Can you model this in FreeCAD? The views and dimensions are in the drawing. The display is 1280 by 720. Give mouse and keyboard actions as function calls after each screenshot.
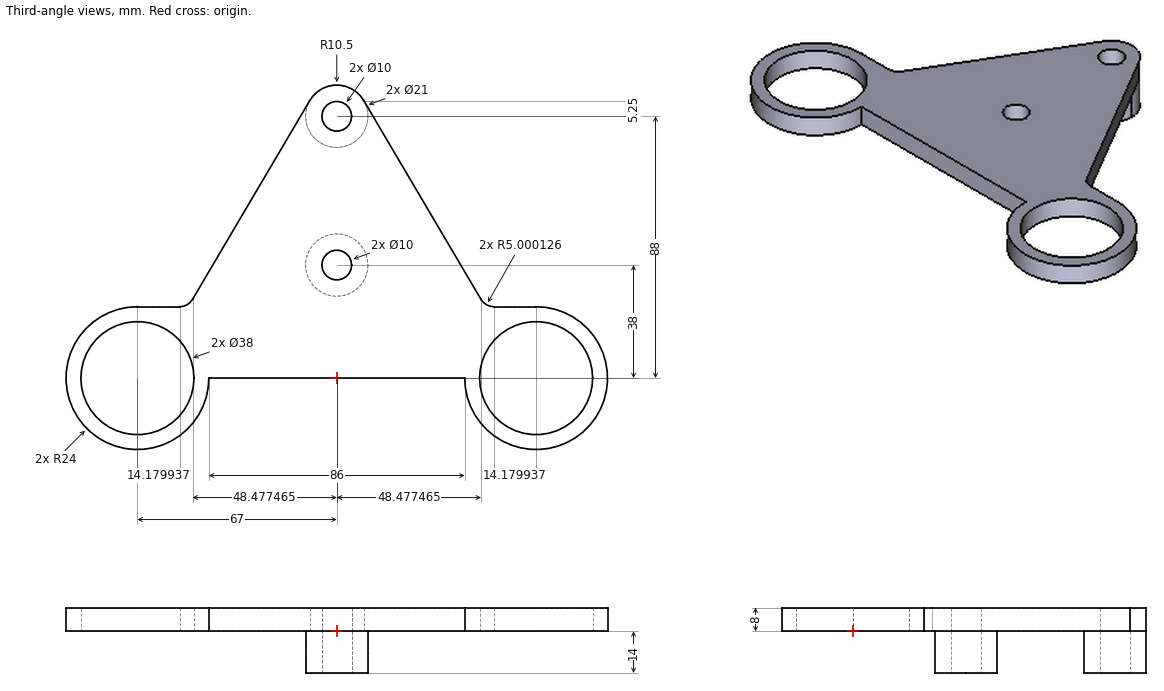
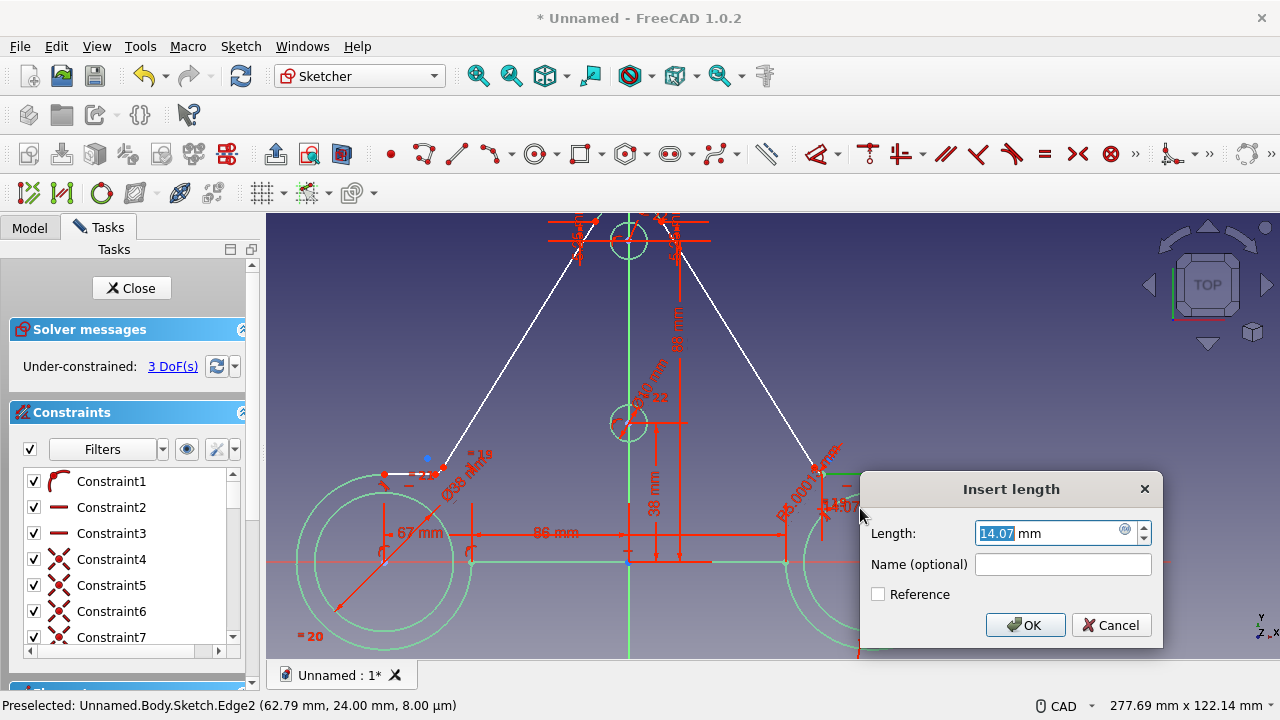
text(14.179937)
key(Return)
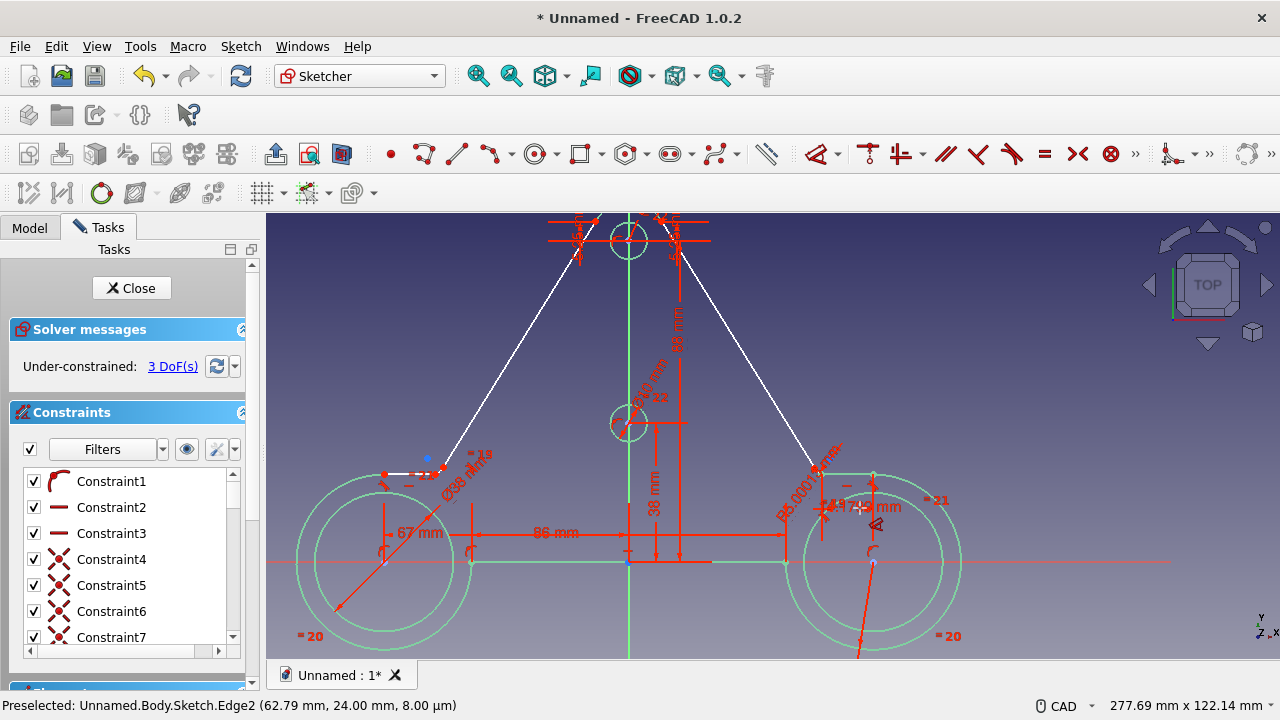
click(420, 474)
click(398, 508)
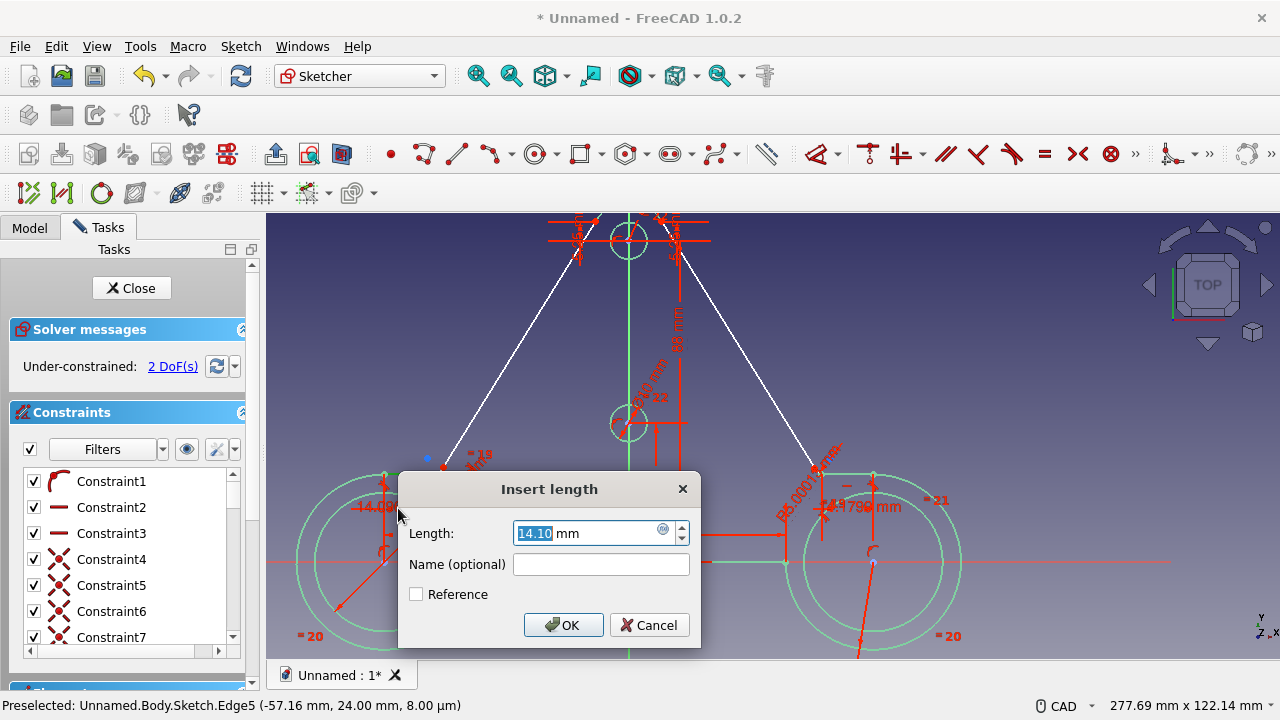
text(14.179937)
key(Return)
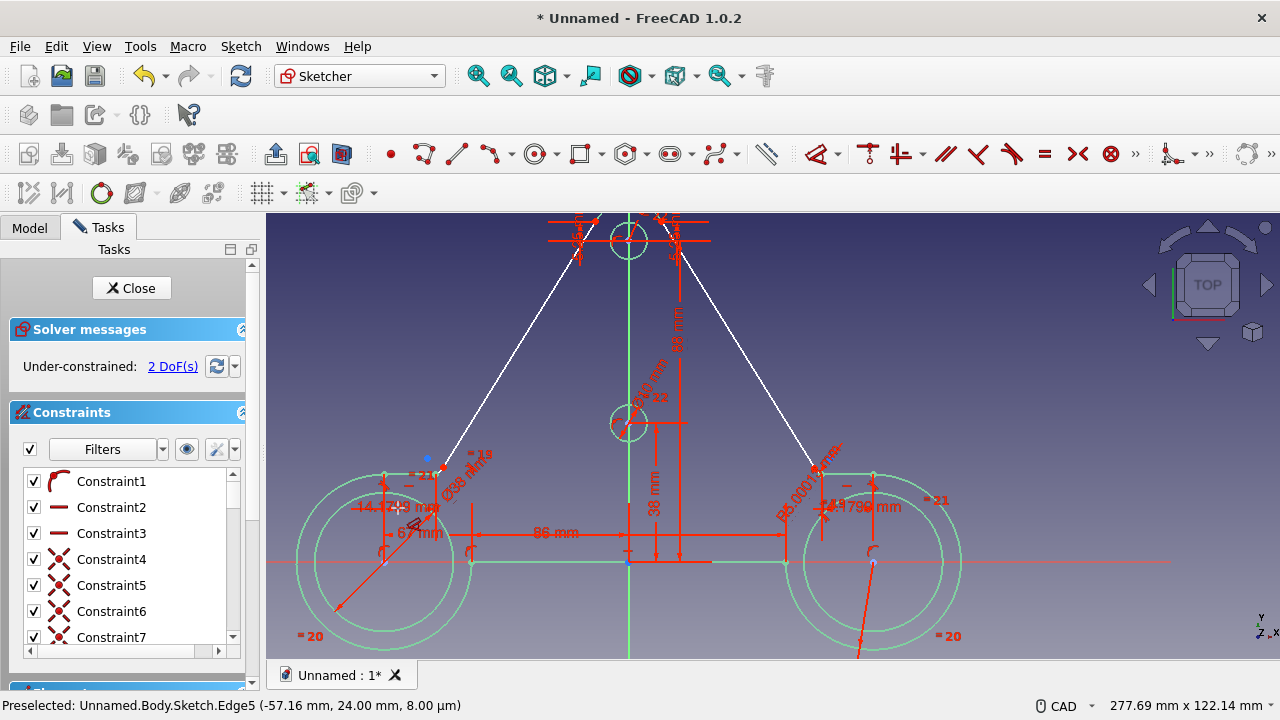
scroll(815, 468, up, 2)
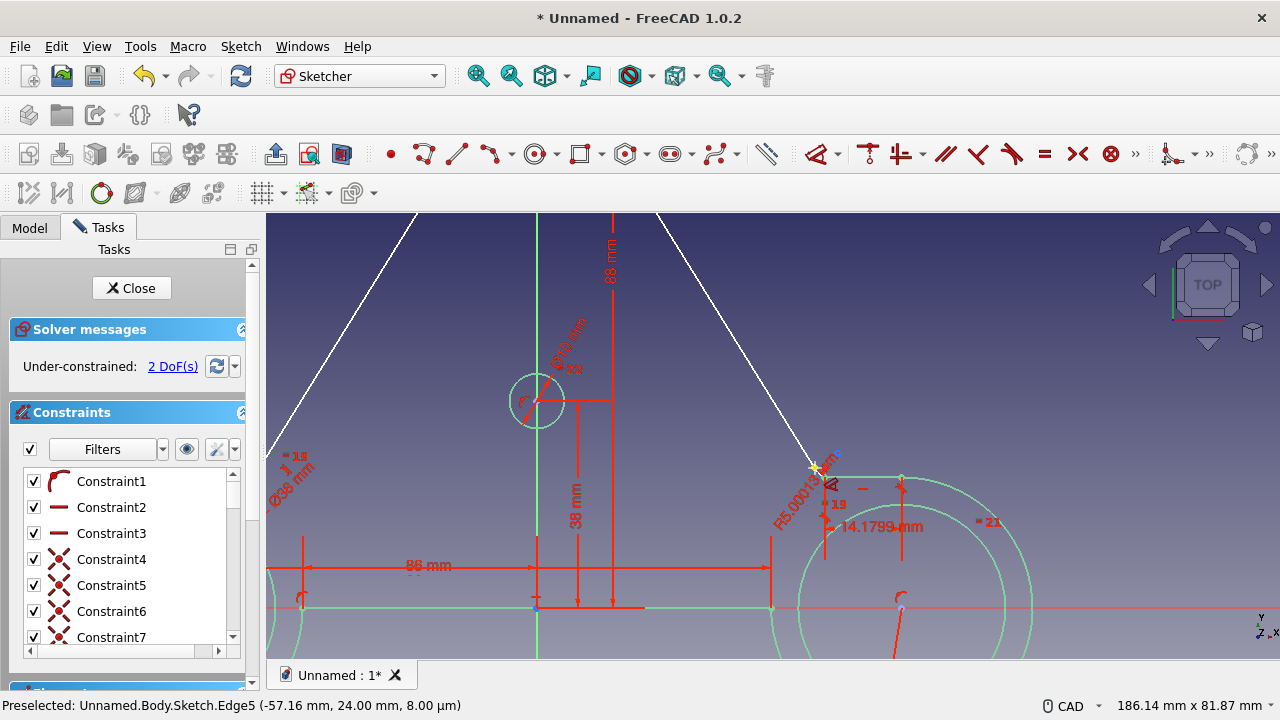
click(815, 468)
click(676, 434)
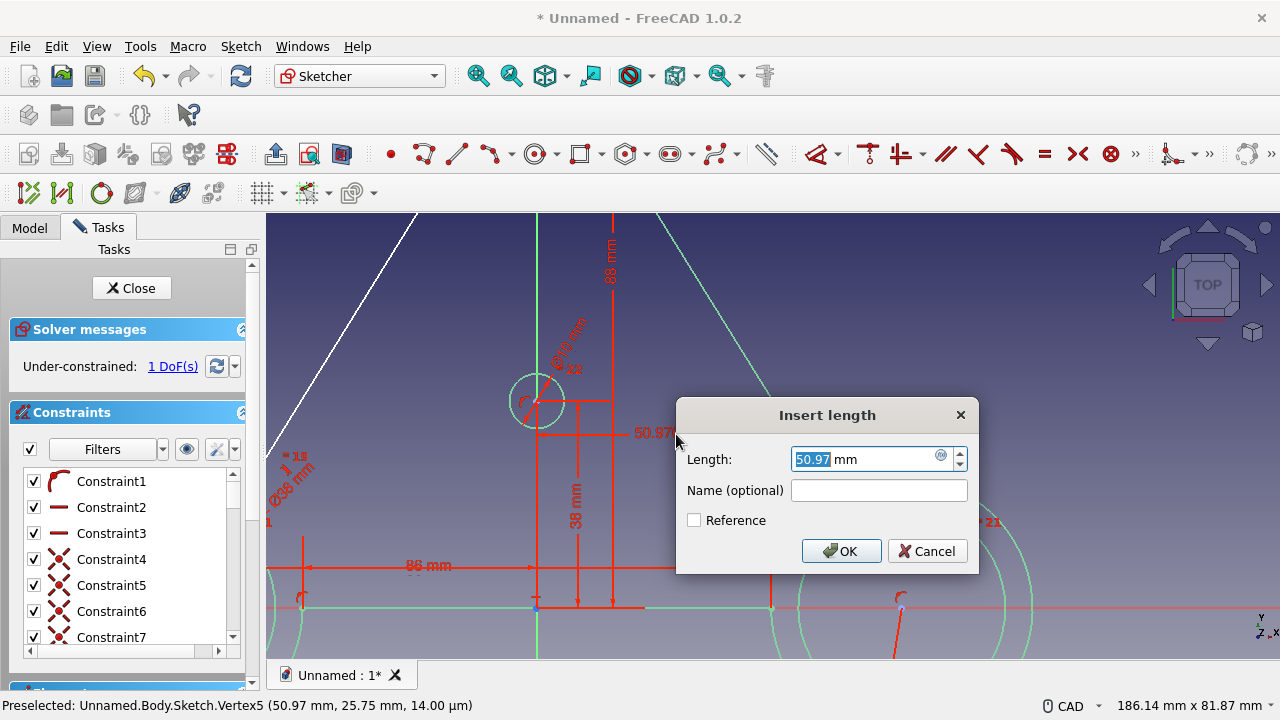
text(48.477465)
key(Return)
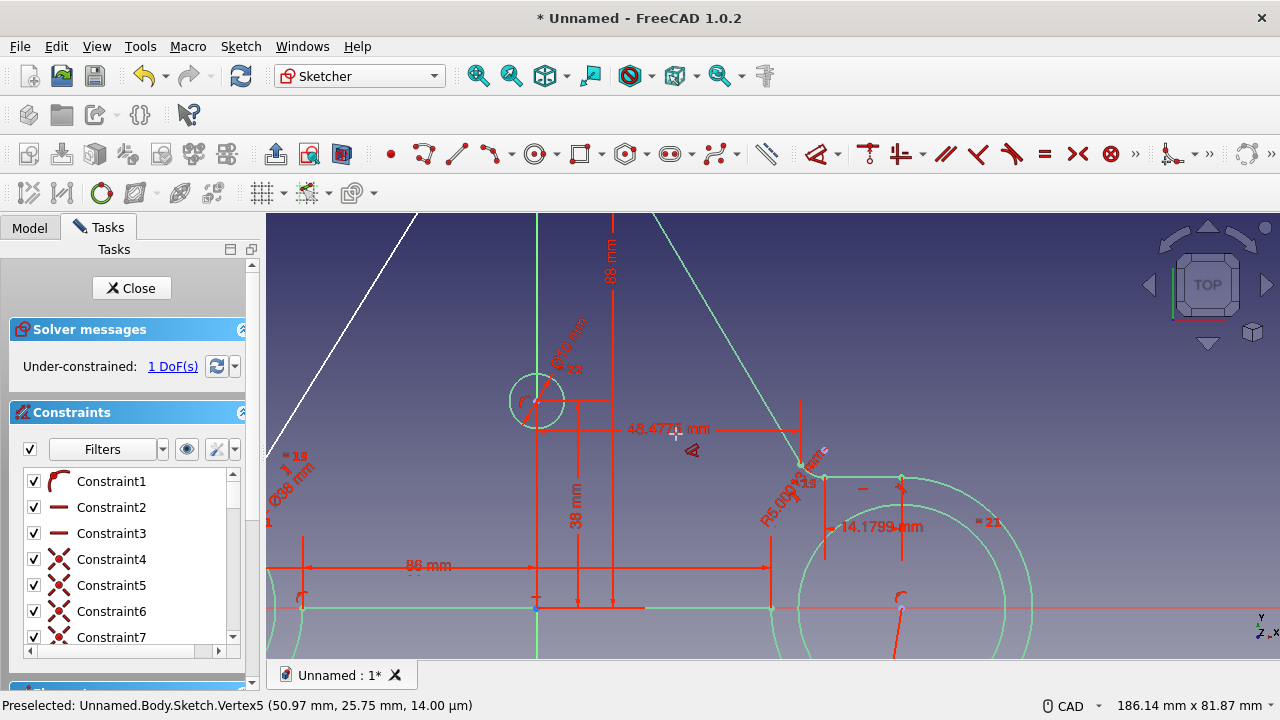
scroll(841, 472, down, 4)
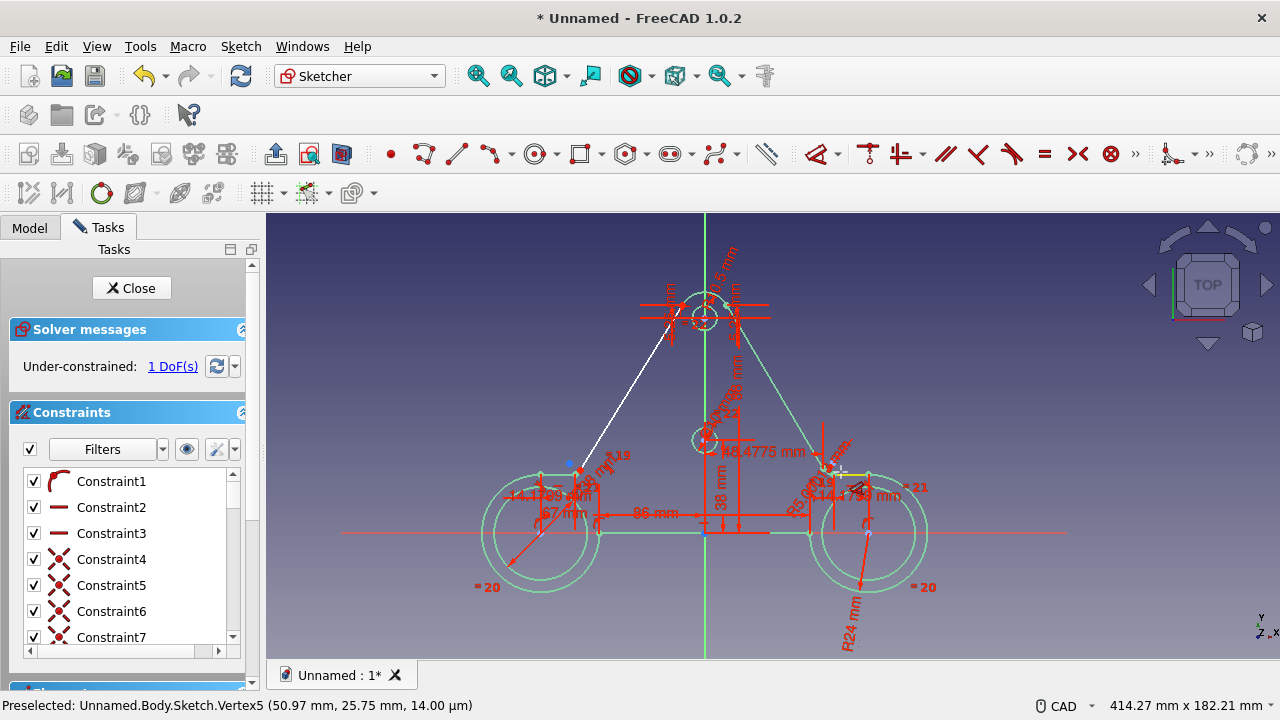
scroll(580, 470, up, 4)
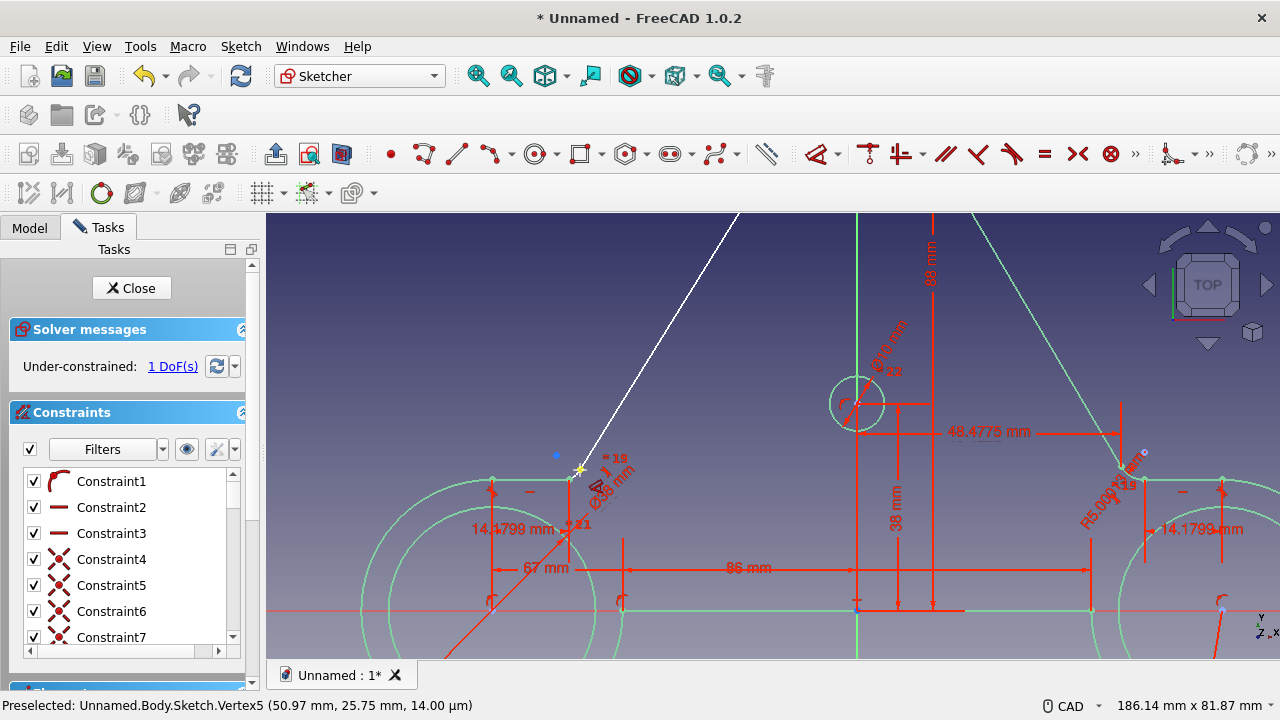
click(580, 470)
click(719, 436)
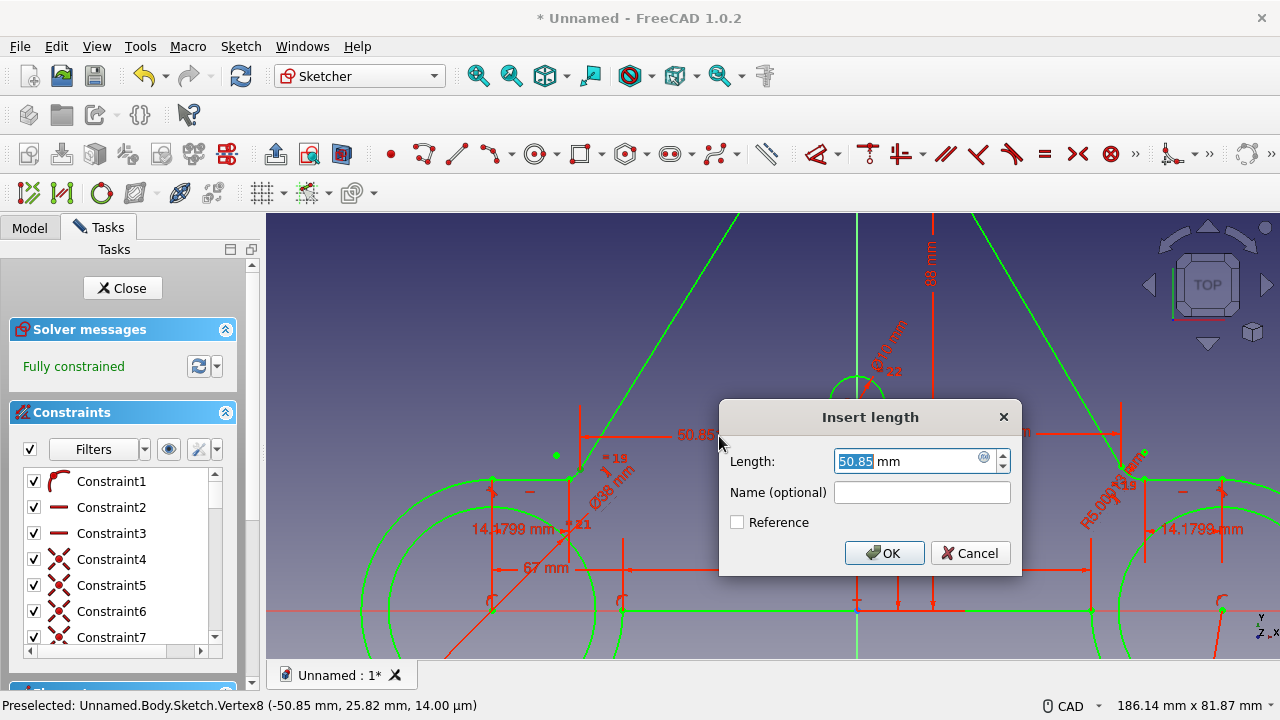
text(48.477465)
key(Return)
key(Escape)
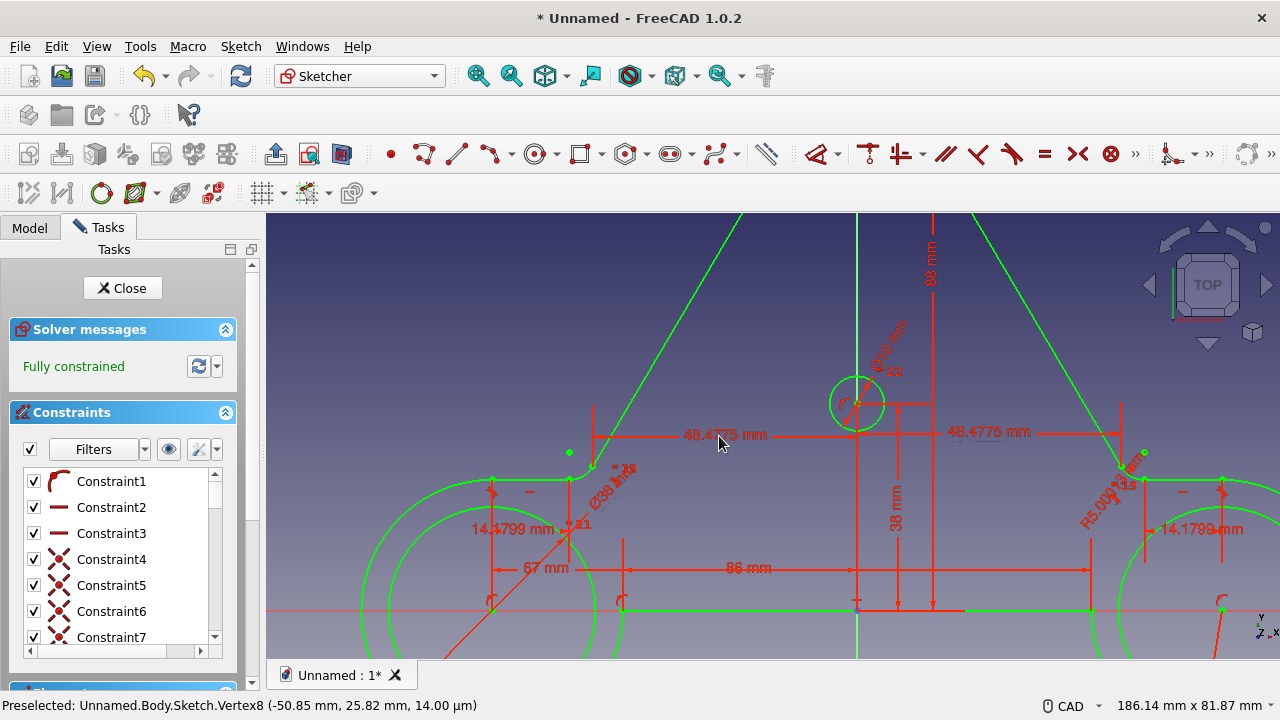
click(123, 288)